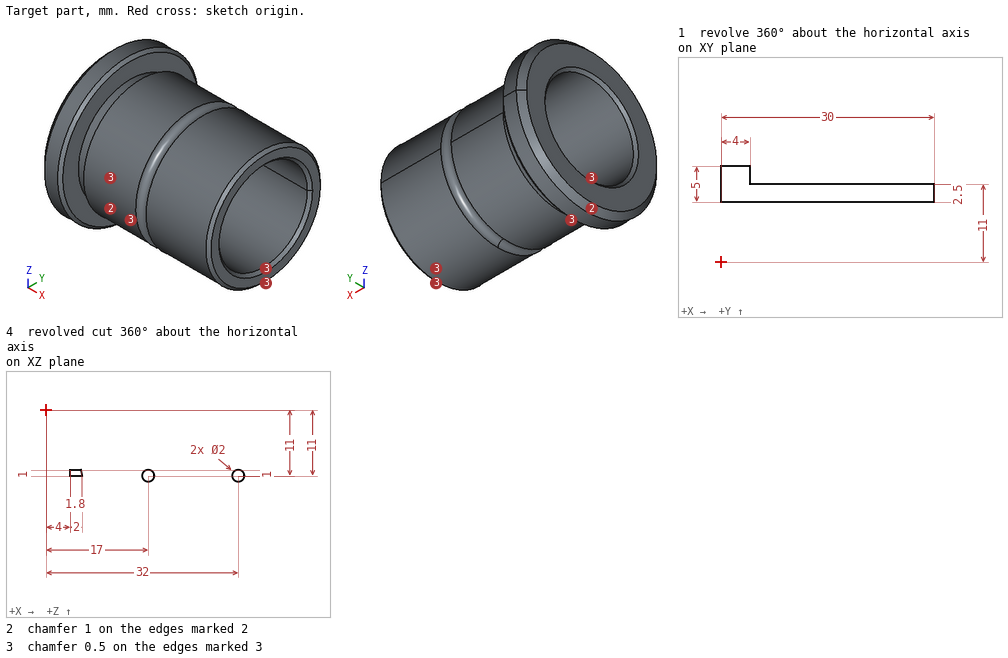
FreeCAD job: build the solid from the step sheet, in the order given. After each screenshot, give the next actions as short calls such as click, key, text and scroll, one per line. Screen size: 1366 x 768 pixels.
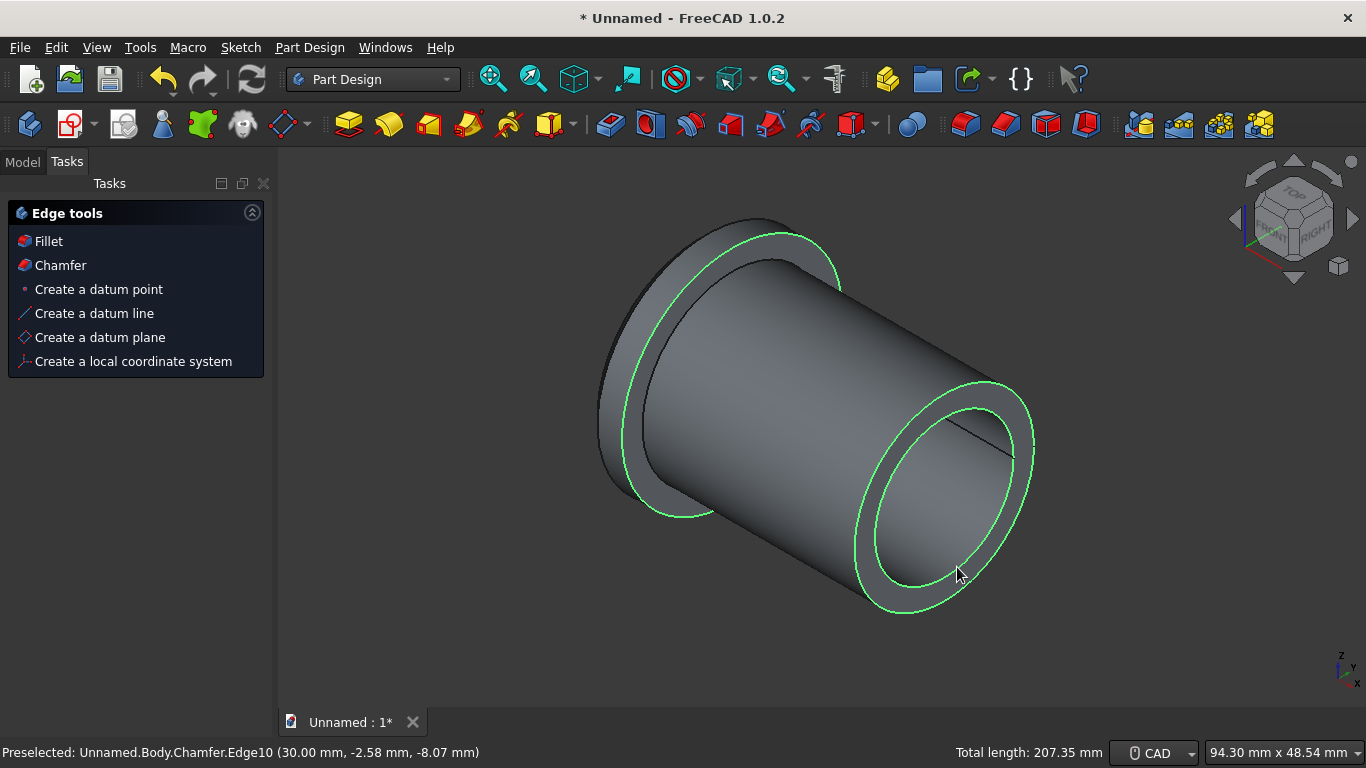
key(2)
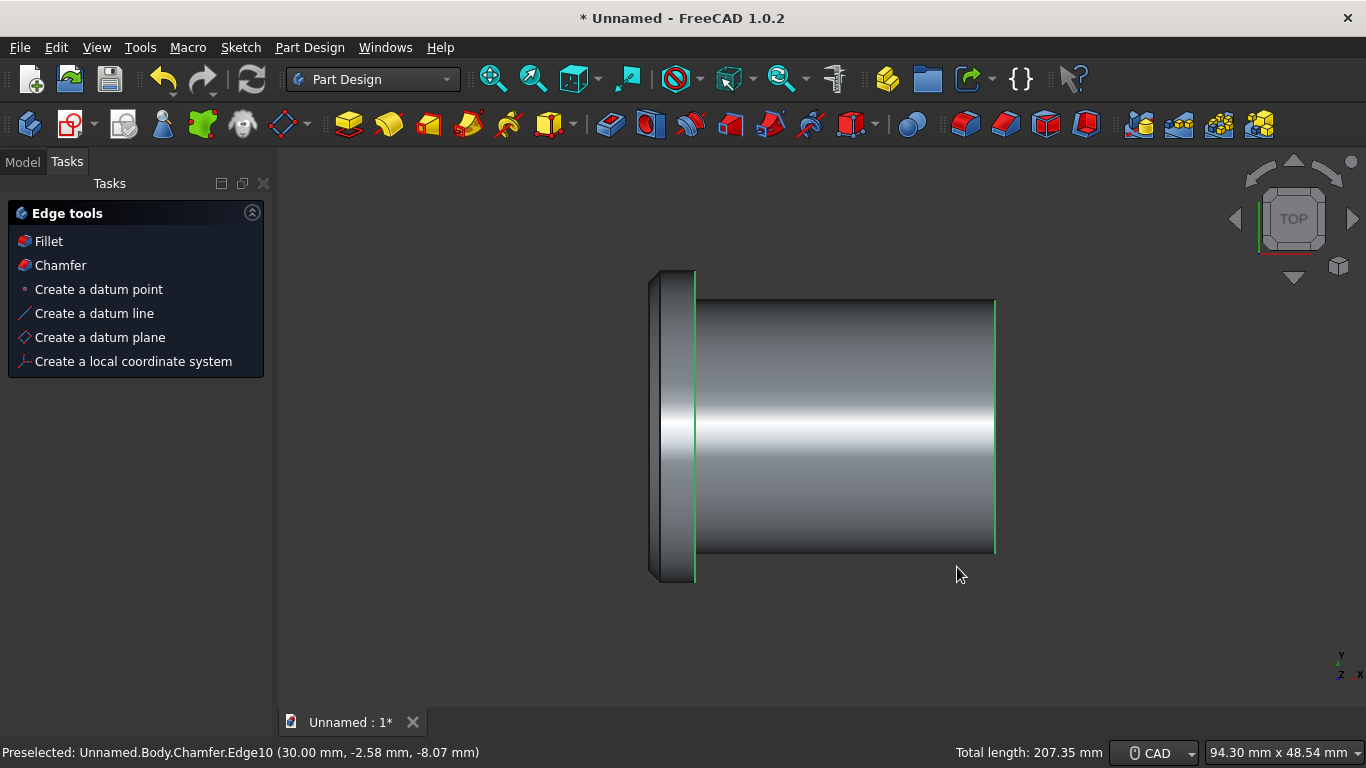
key(1)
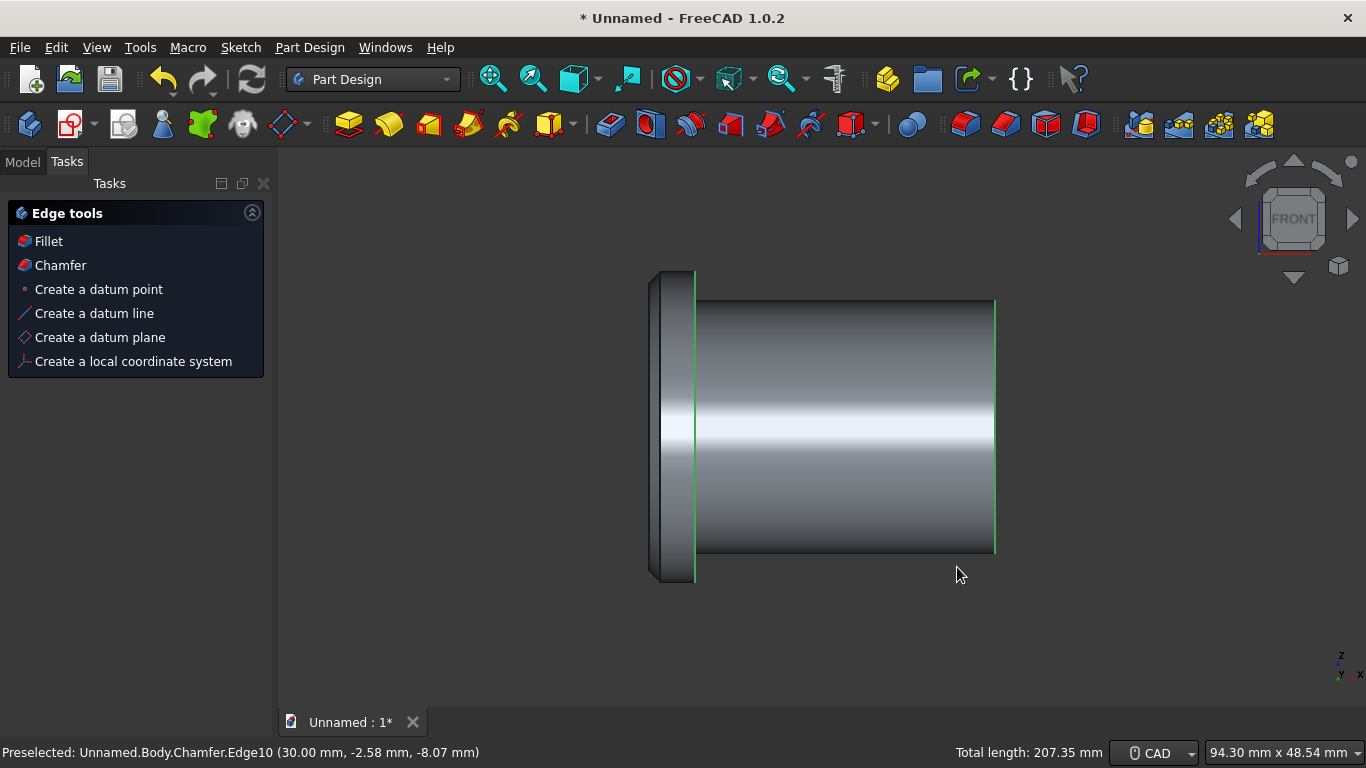
key(3)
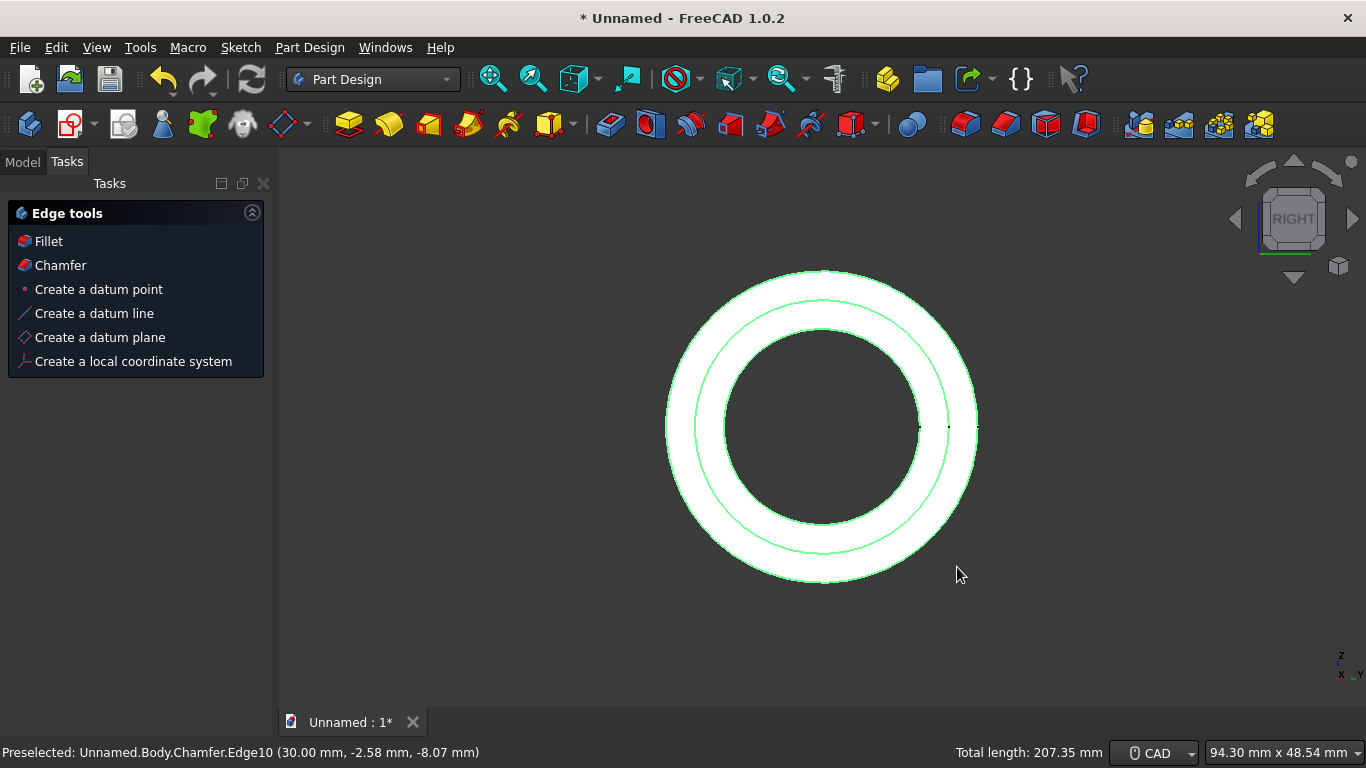
key(5)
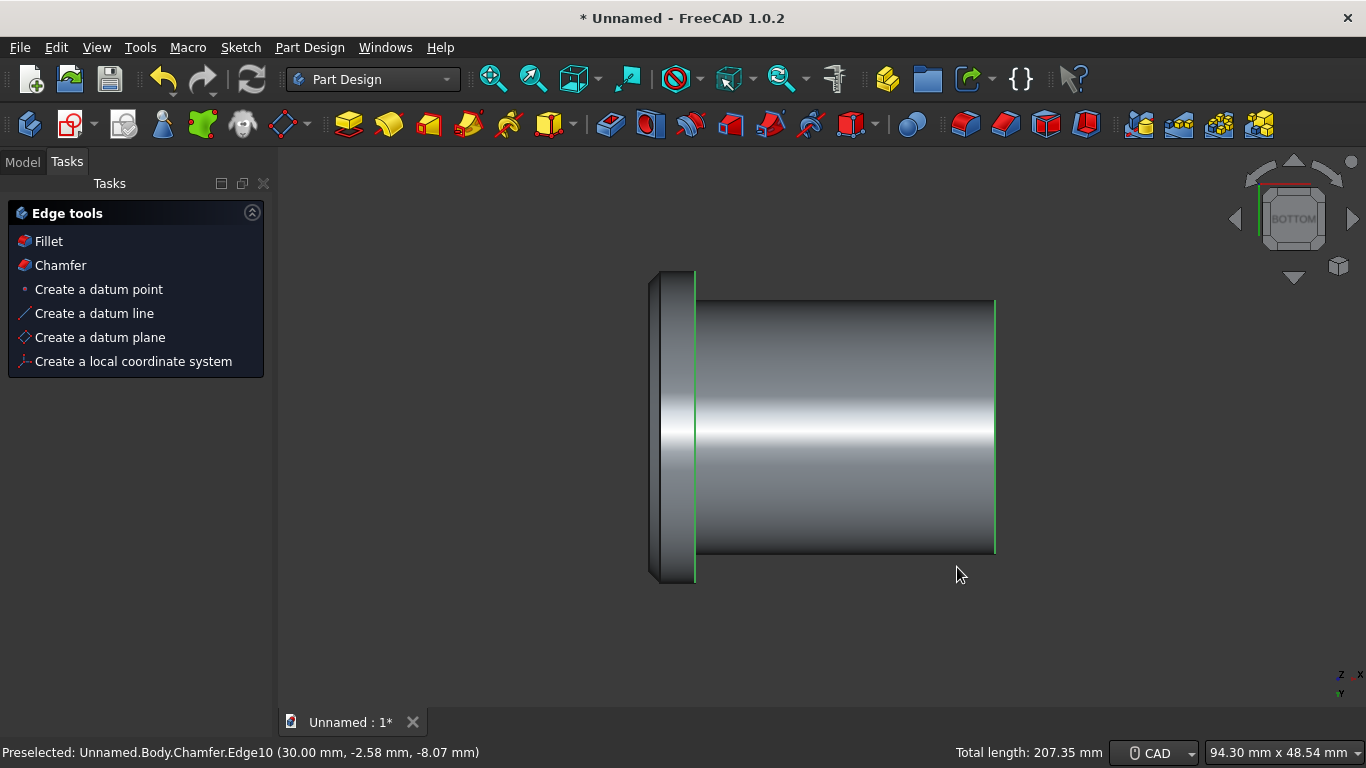
key(4)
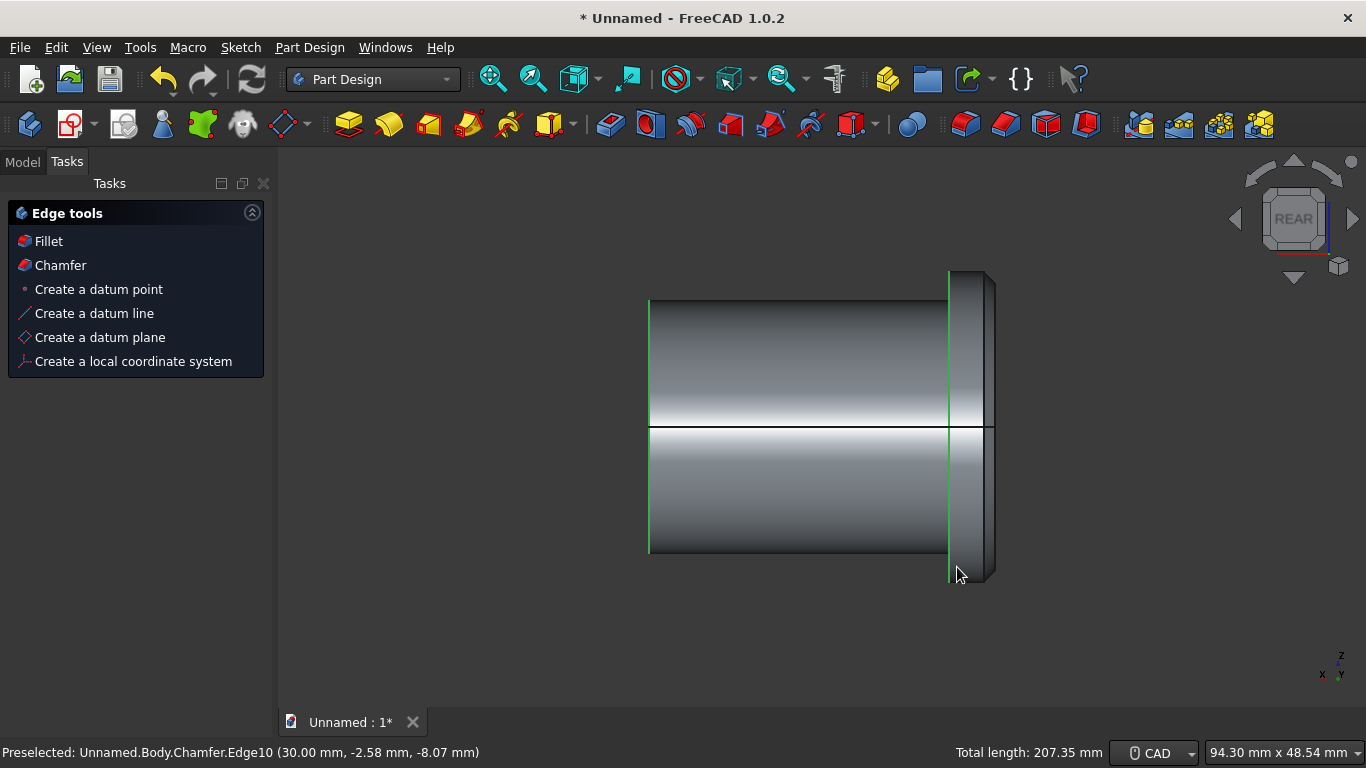
key(6)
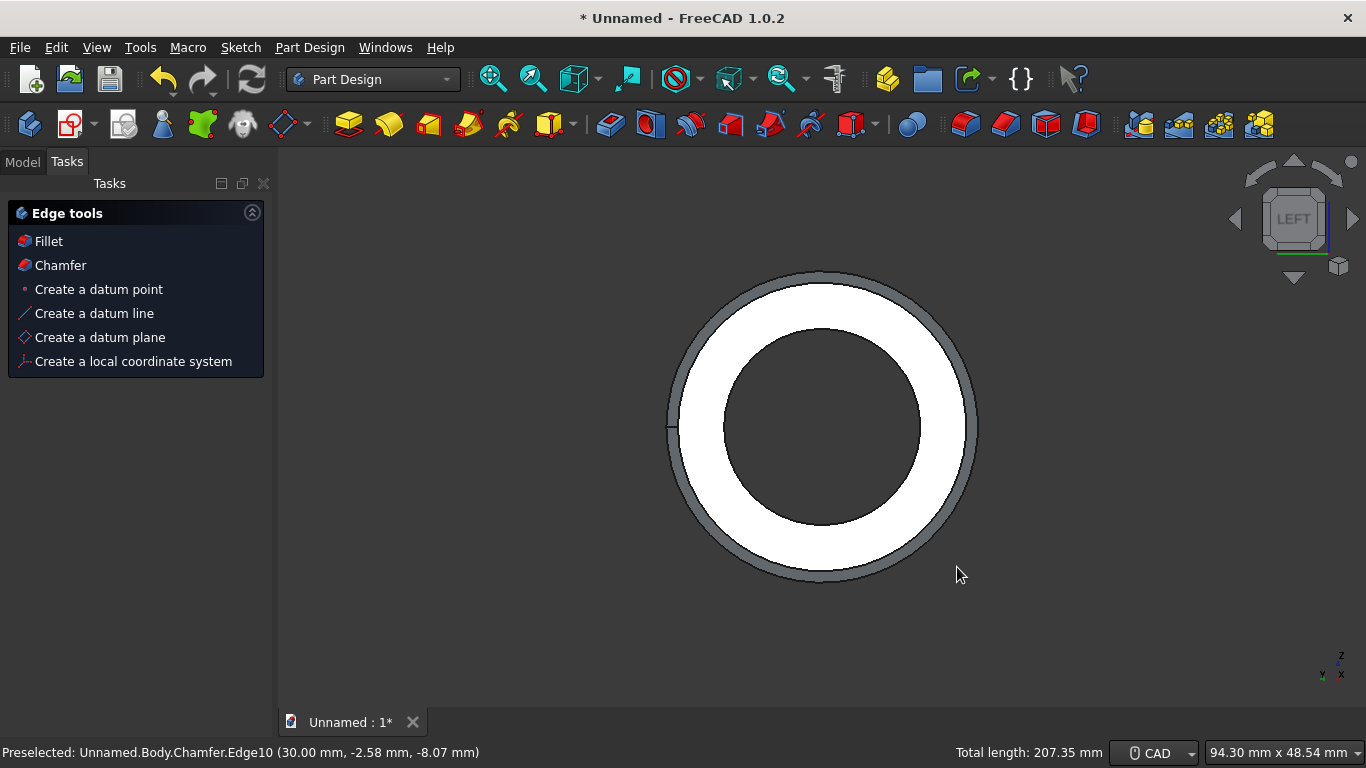
click(920, 426, ctrl)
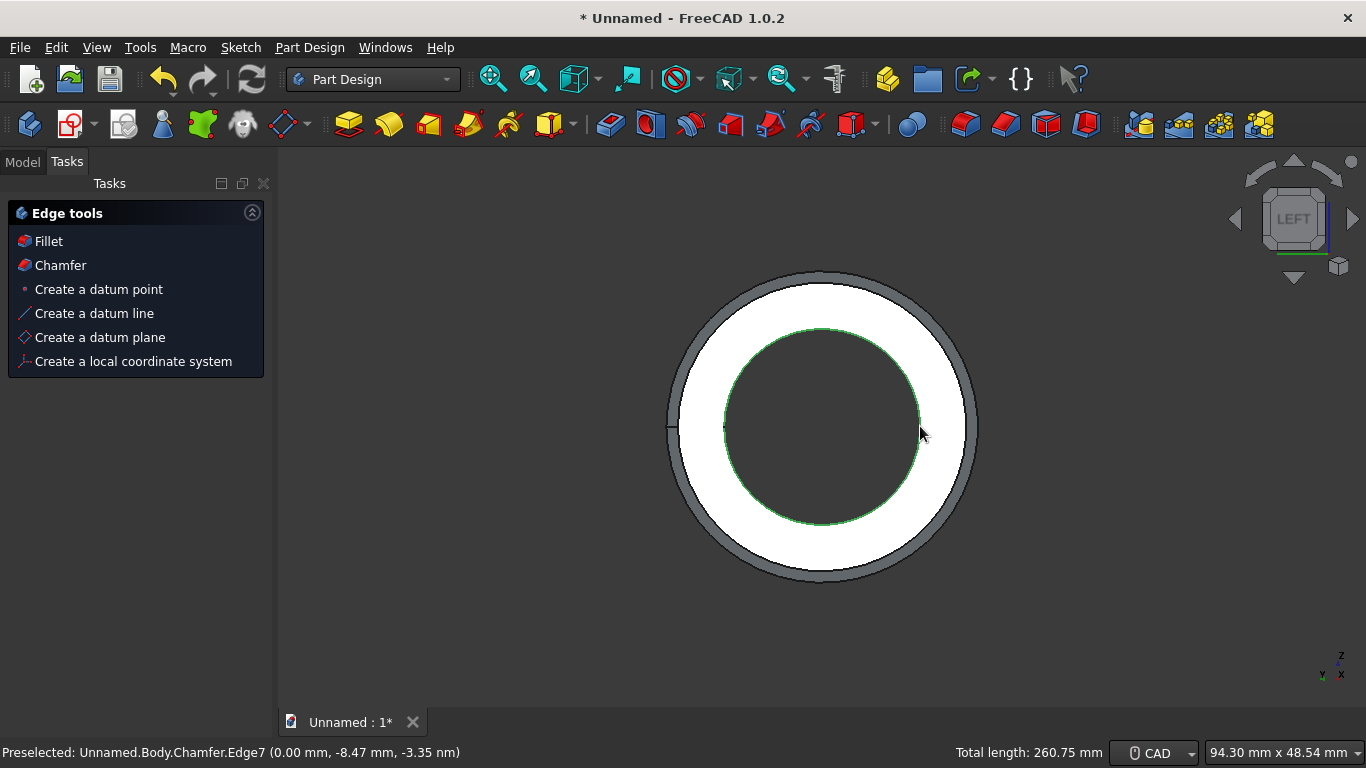
click(1006, 124)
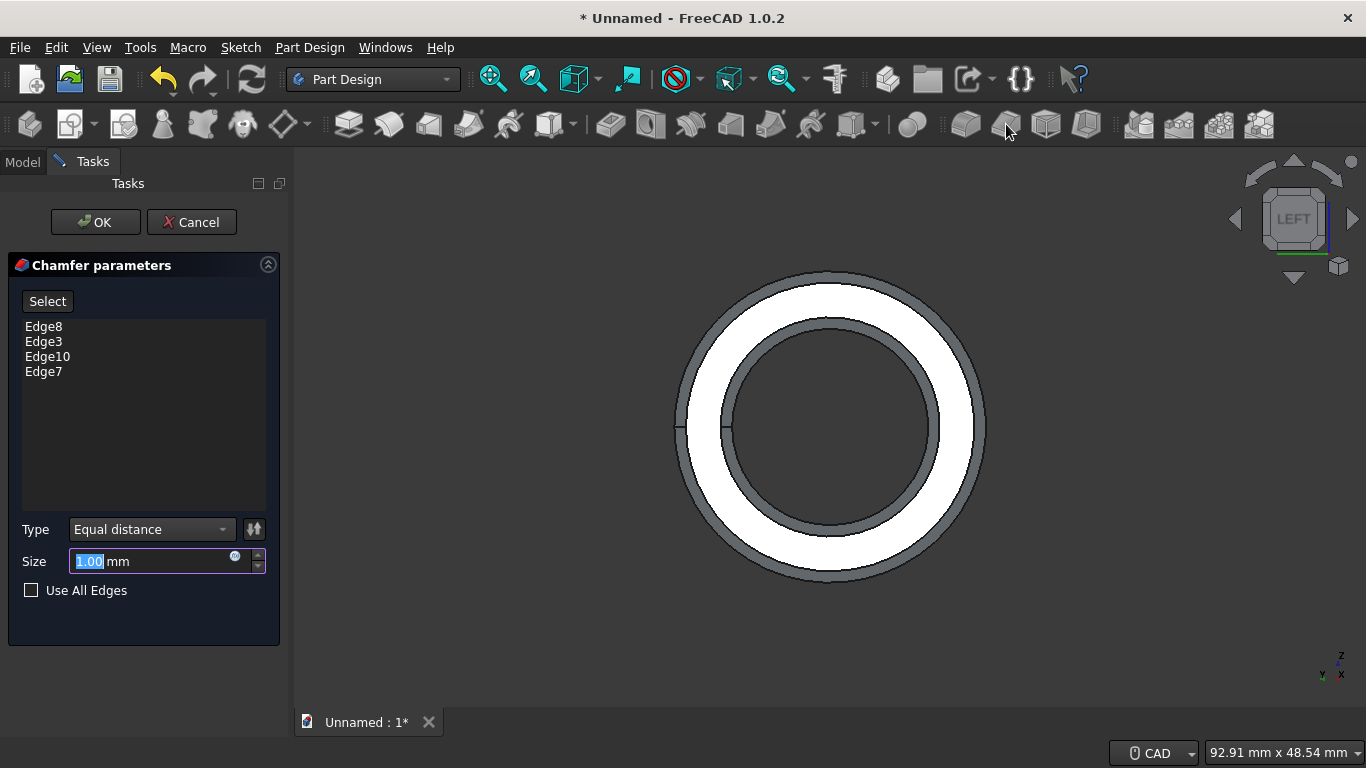
text(0.5)
key(Tab)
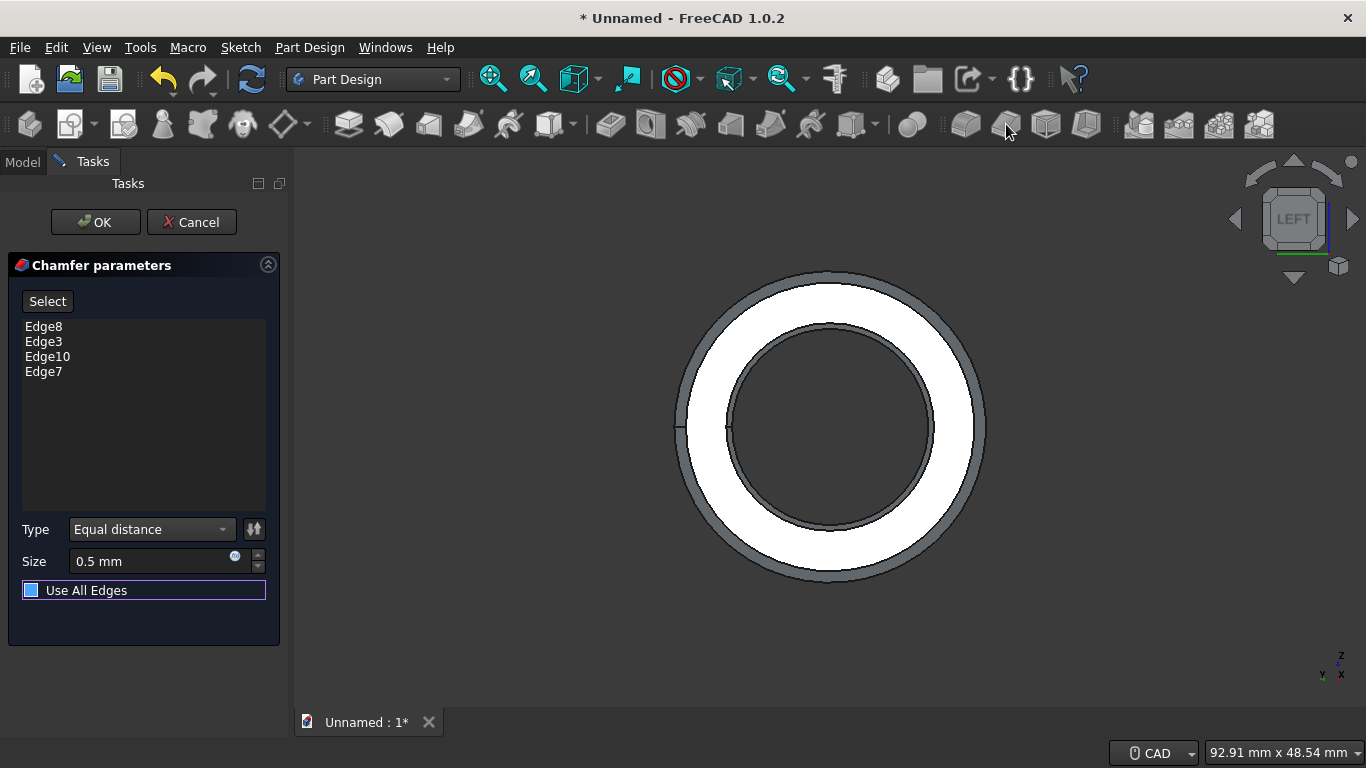
click(96, 222)